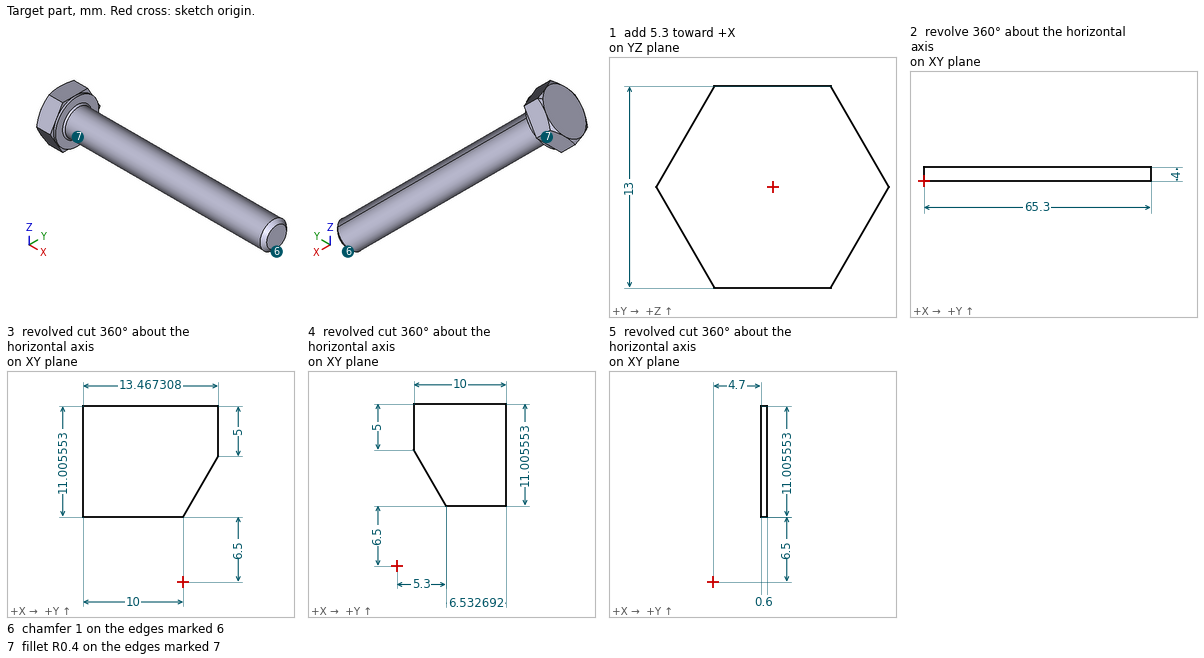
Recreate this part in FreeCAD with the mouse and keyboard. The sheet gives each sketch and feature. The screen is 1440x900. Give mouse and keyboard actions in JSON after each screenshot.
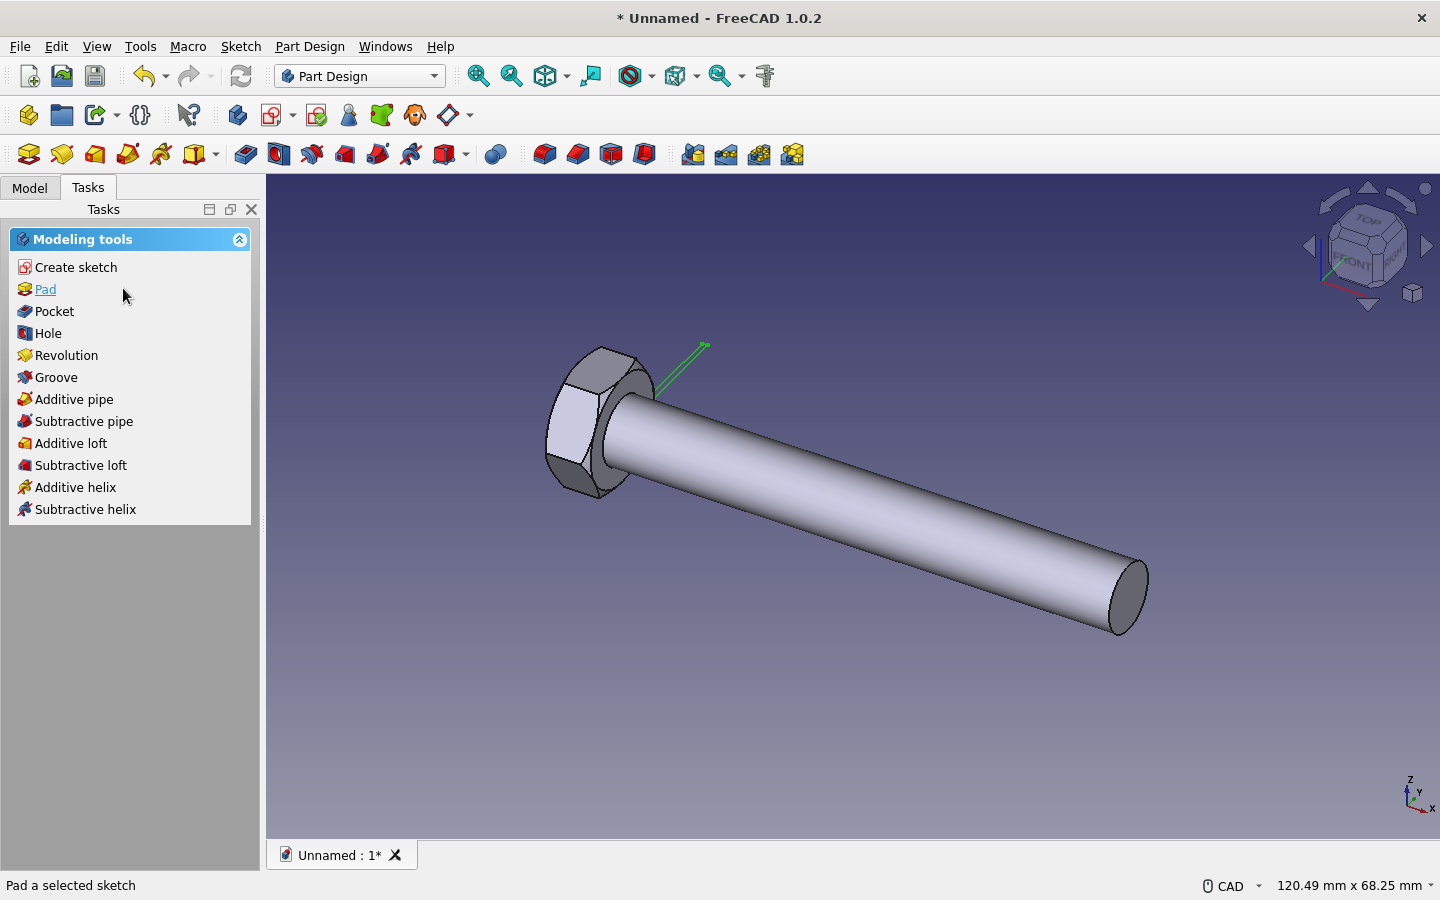
{"action": "left_click", "coordinate": [312, 154]}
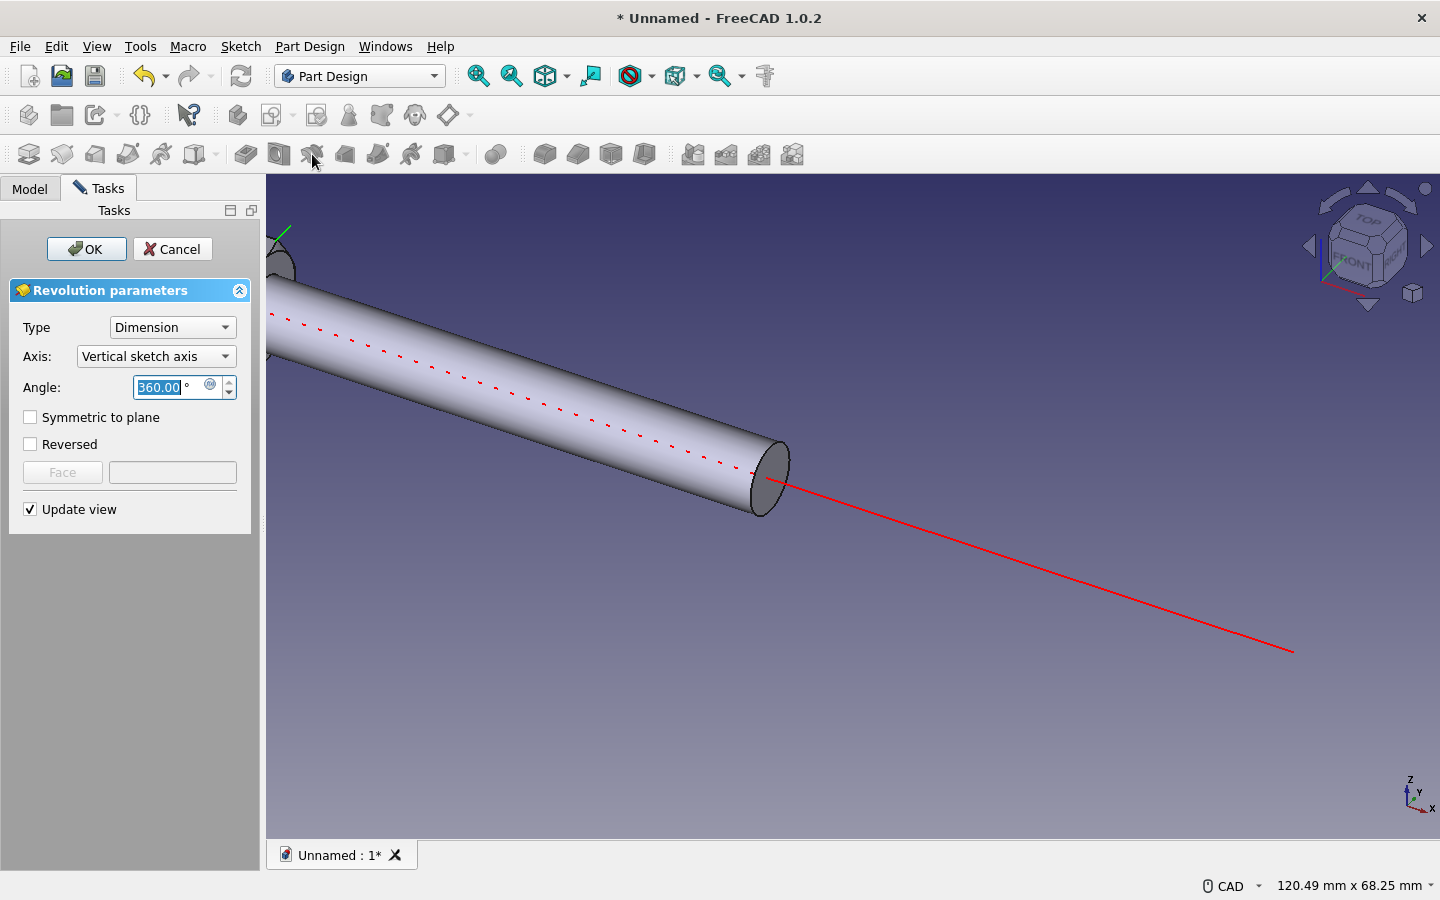
{"action": "left_click", "coordinate": [157, 356]}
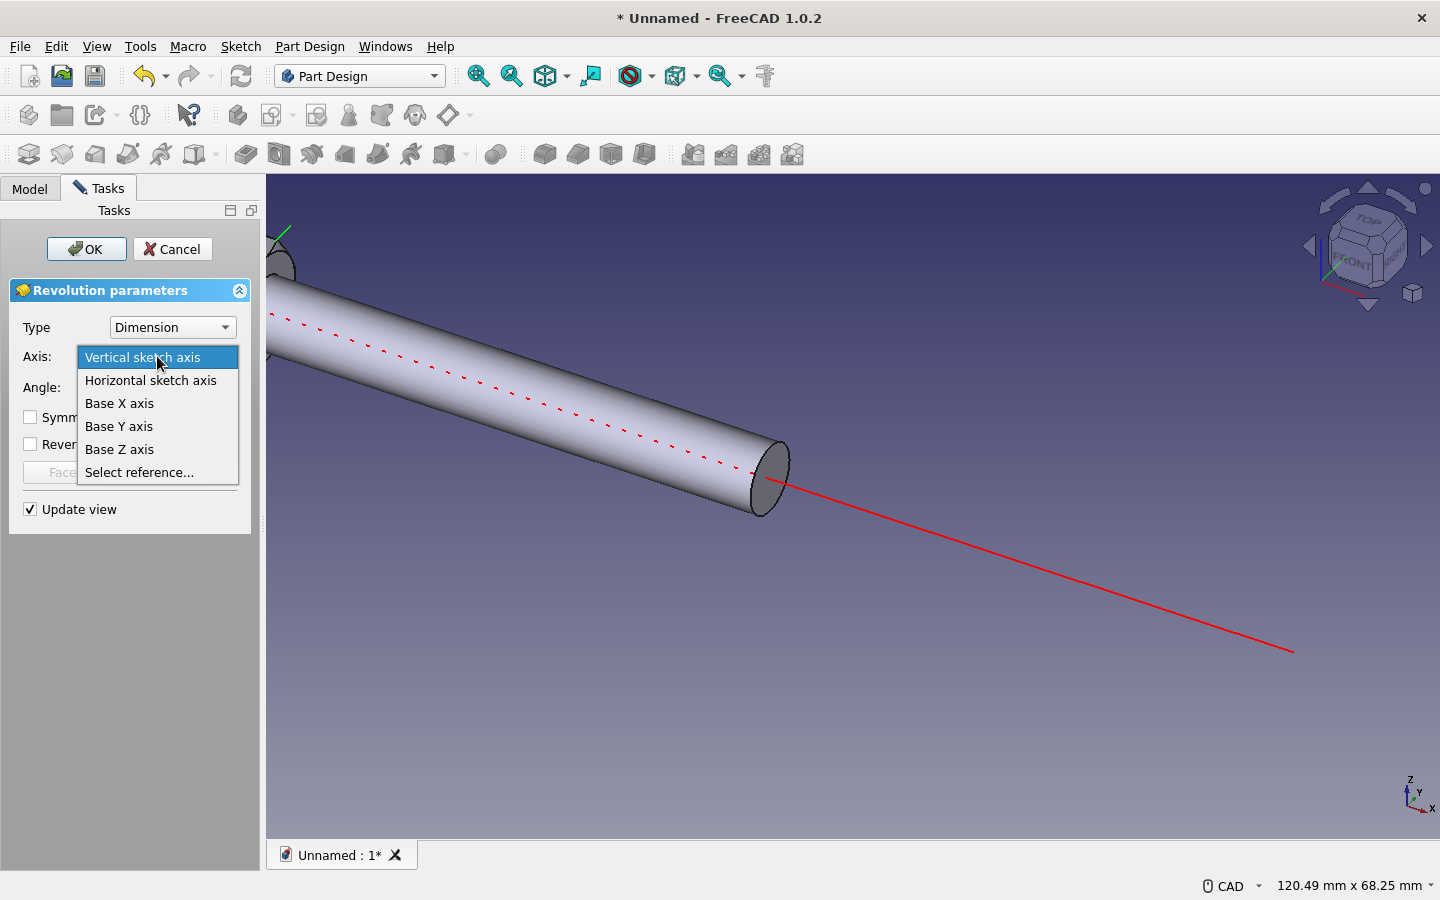
{"action": "left_click", "coordinate": [156, 380]}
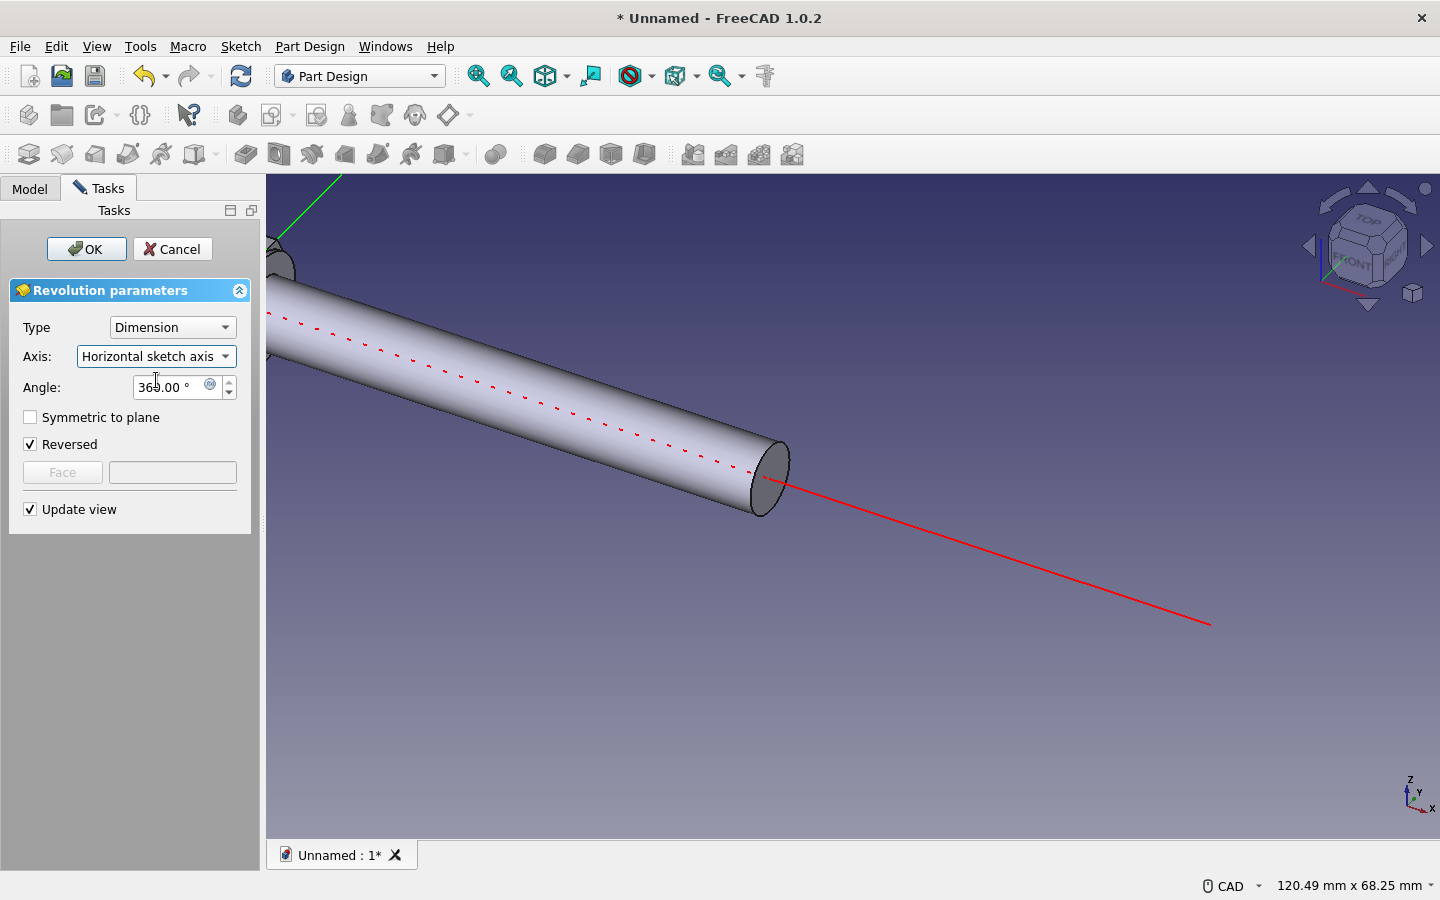
{"action": "left_click", "coordinate": [87, 249]}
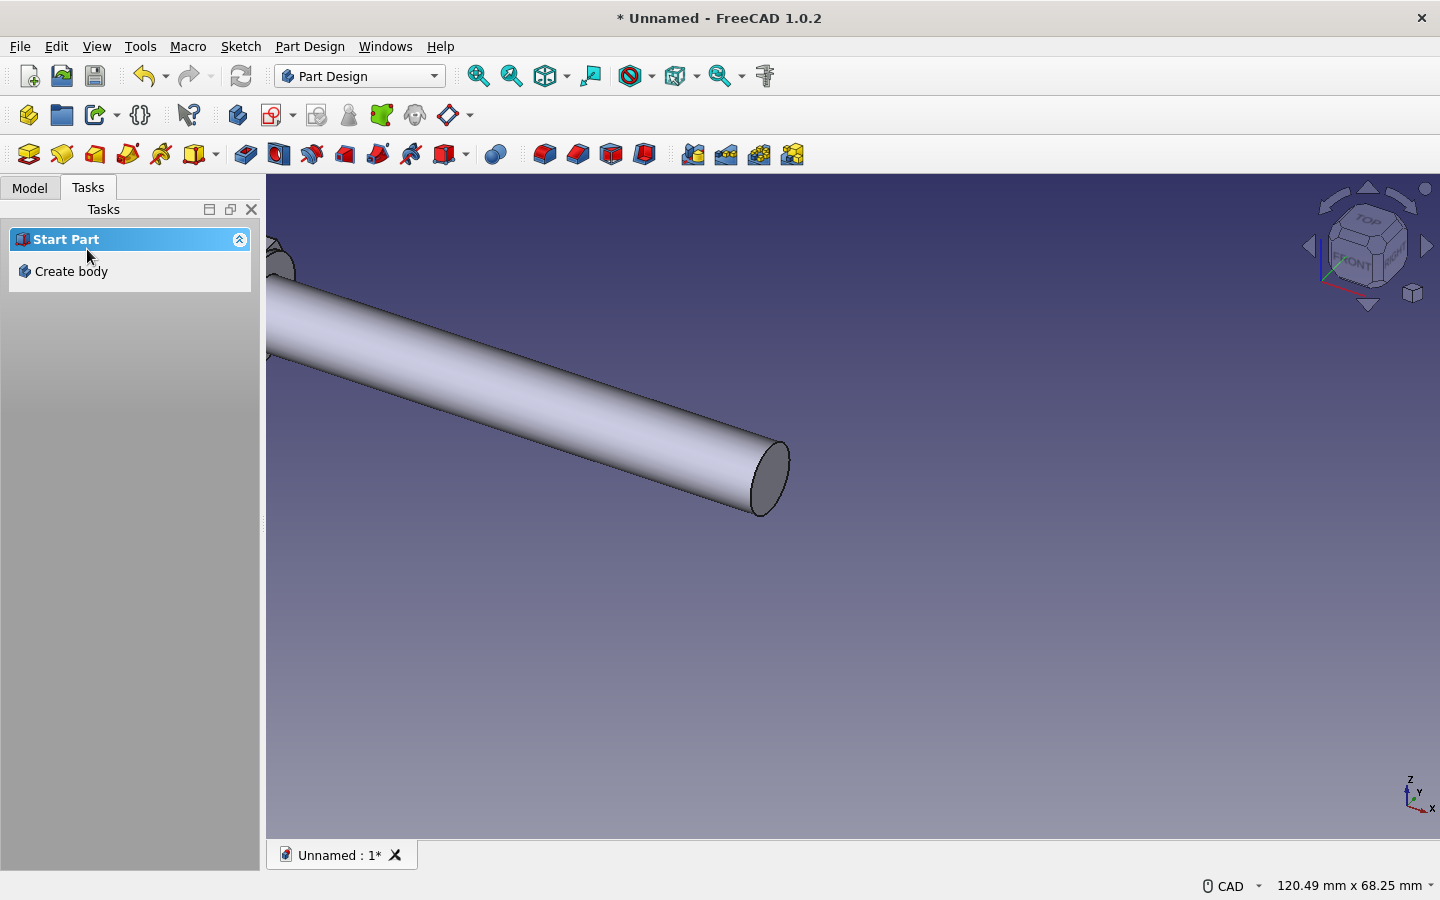
{"action": "left_click", "coordinate": [479, 76]}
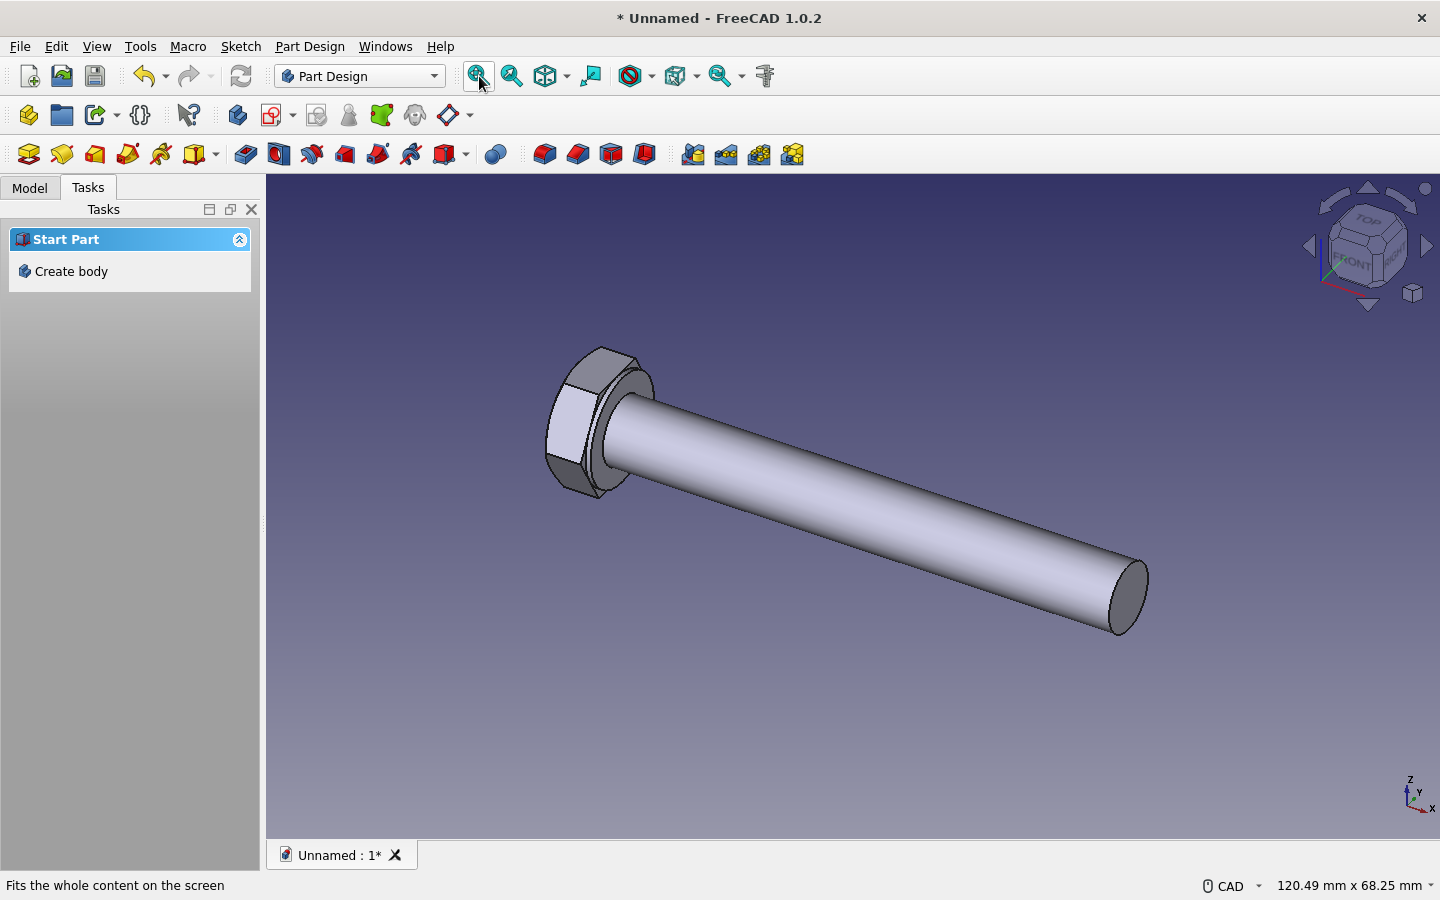
{"action": "left_click", "coordinate": [1109, 616]}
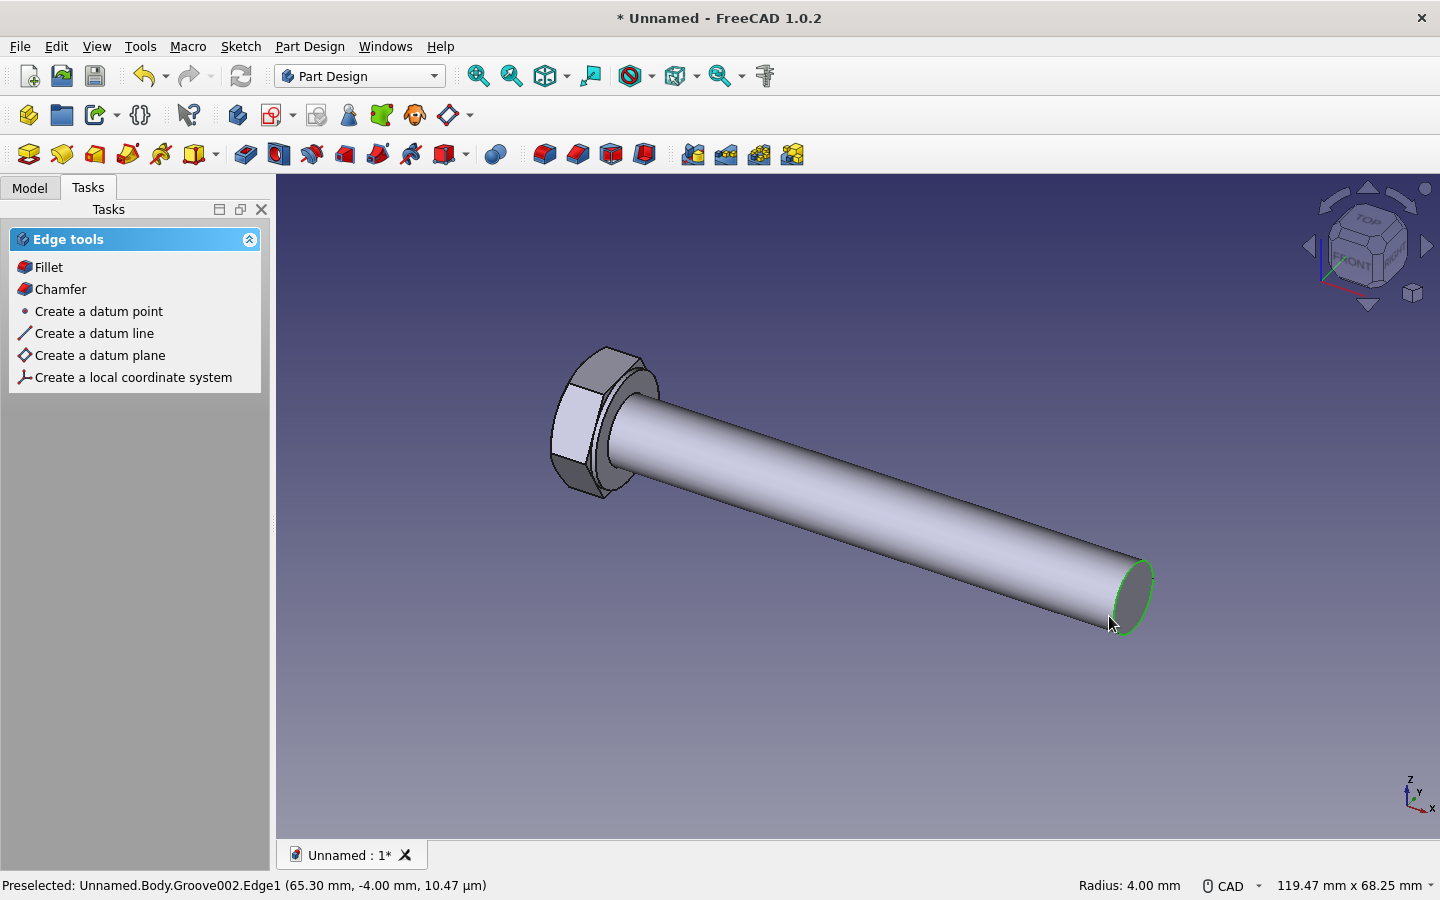
{"action": "left_click", "coordinate": [578, 154]}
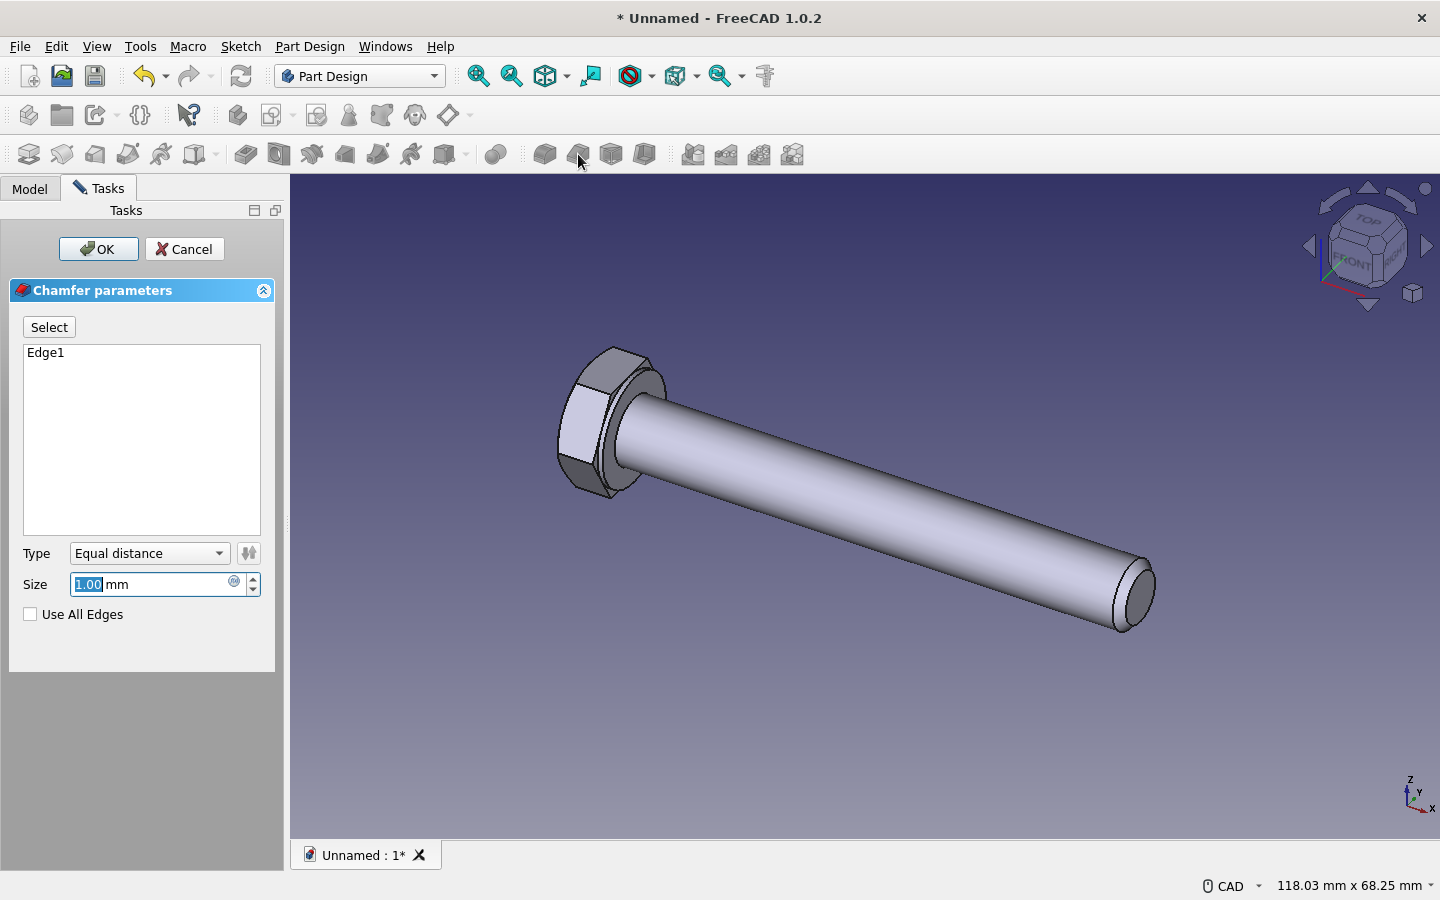
{"action": "type", "text": "1"}
{"action": "key", "text": "Tab"}